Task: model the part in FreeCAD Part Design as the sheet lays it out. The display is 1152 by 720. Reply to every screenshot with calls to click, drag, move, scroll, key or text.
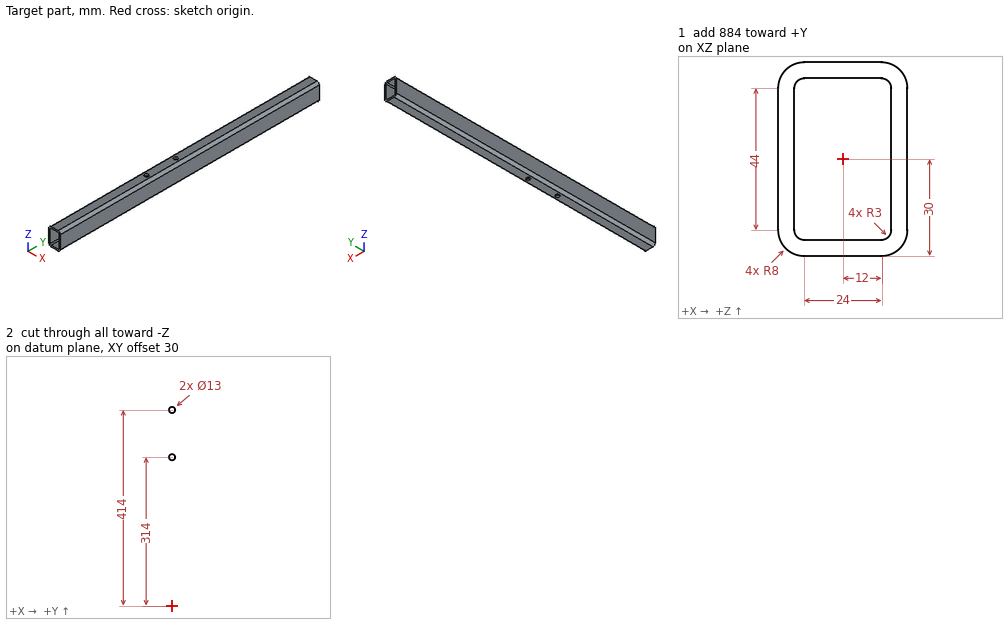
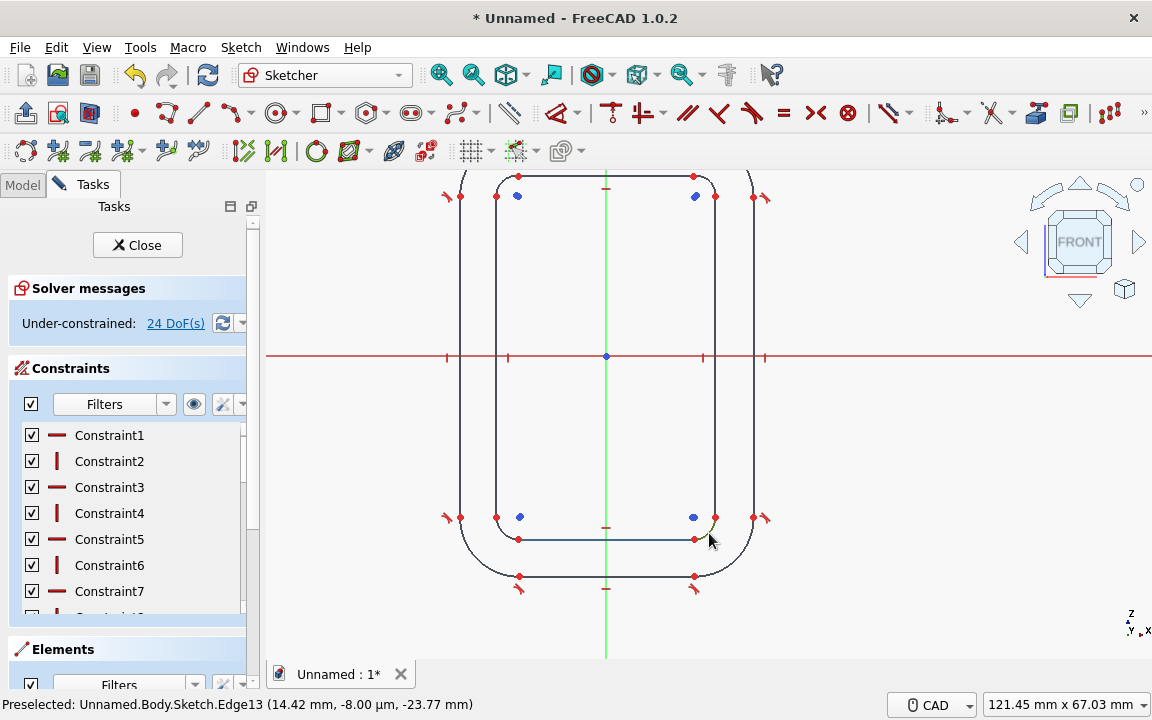
key(t)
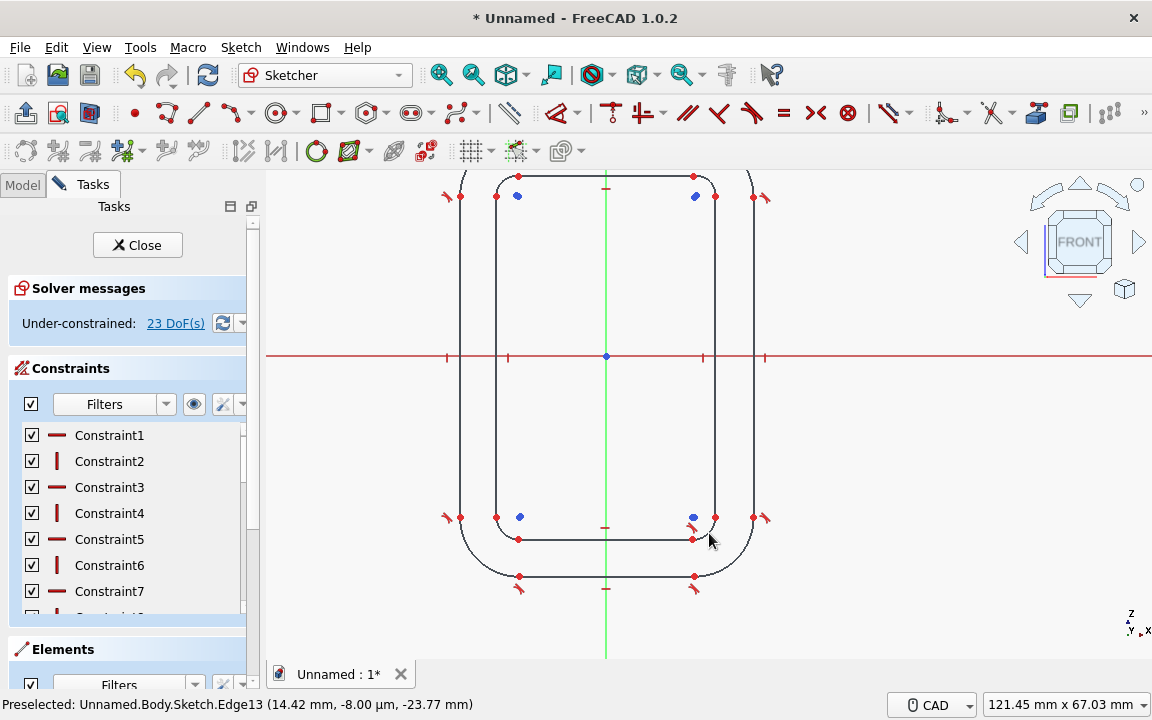
click(571, 540)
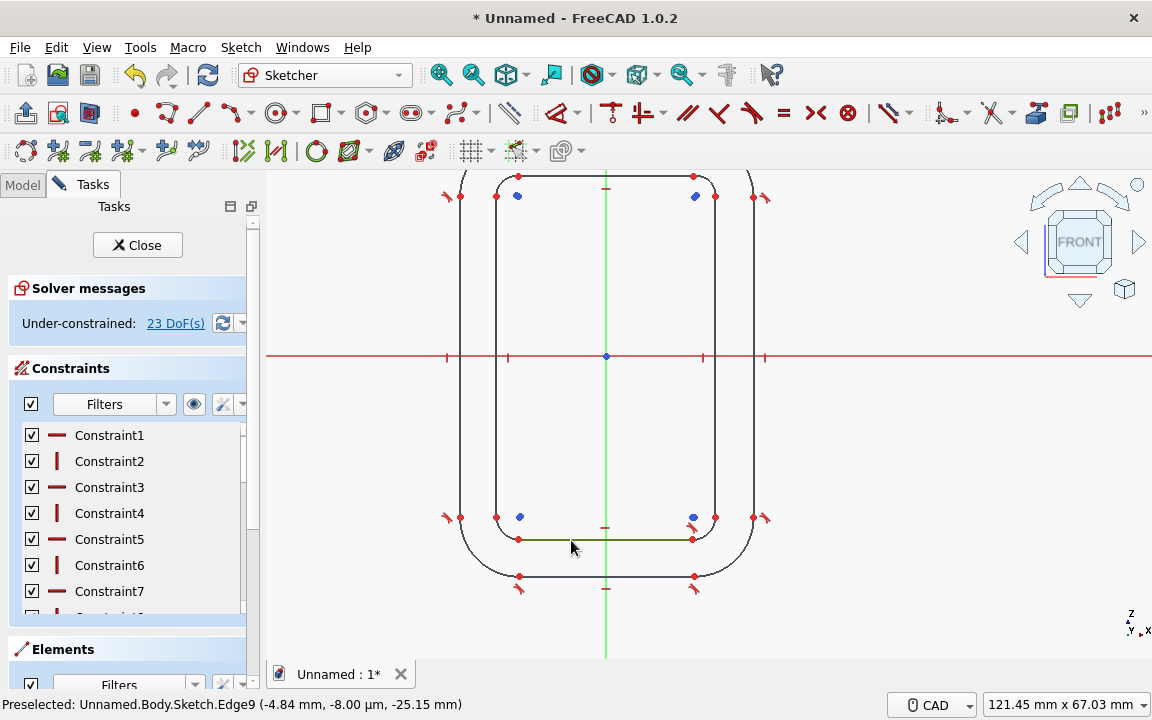
scroll(499, 527, up, 2)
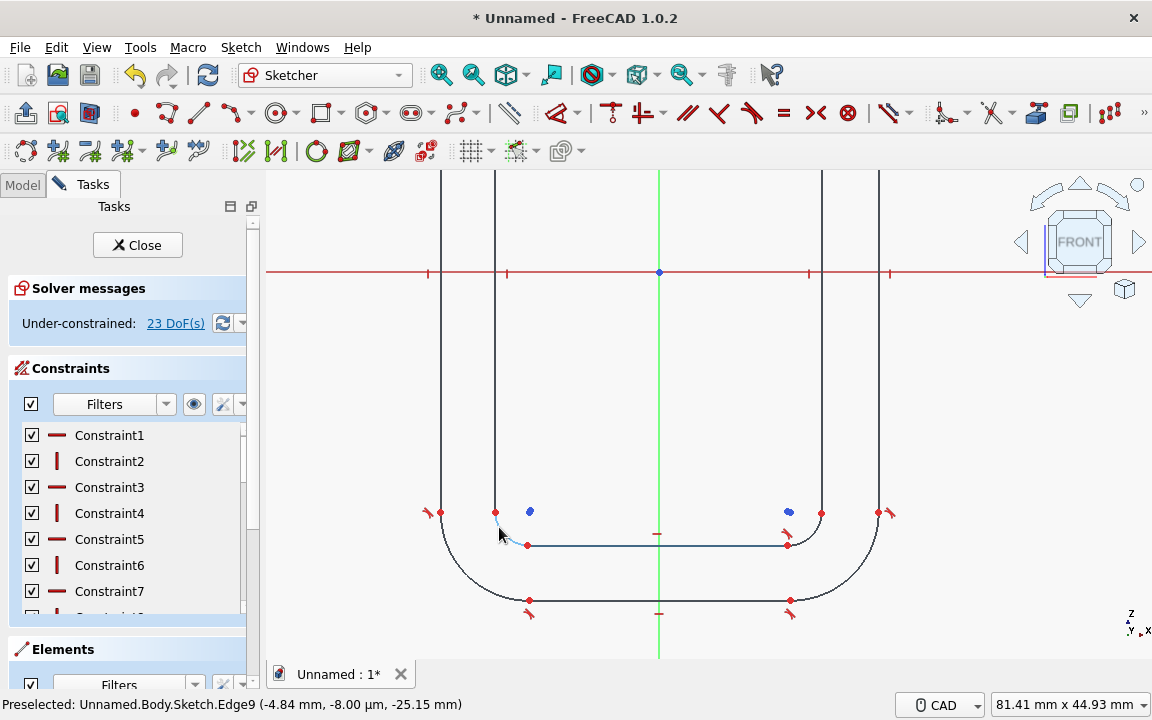
click(499, 527)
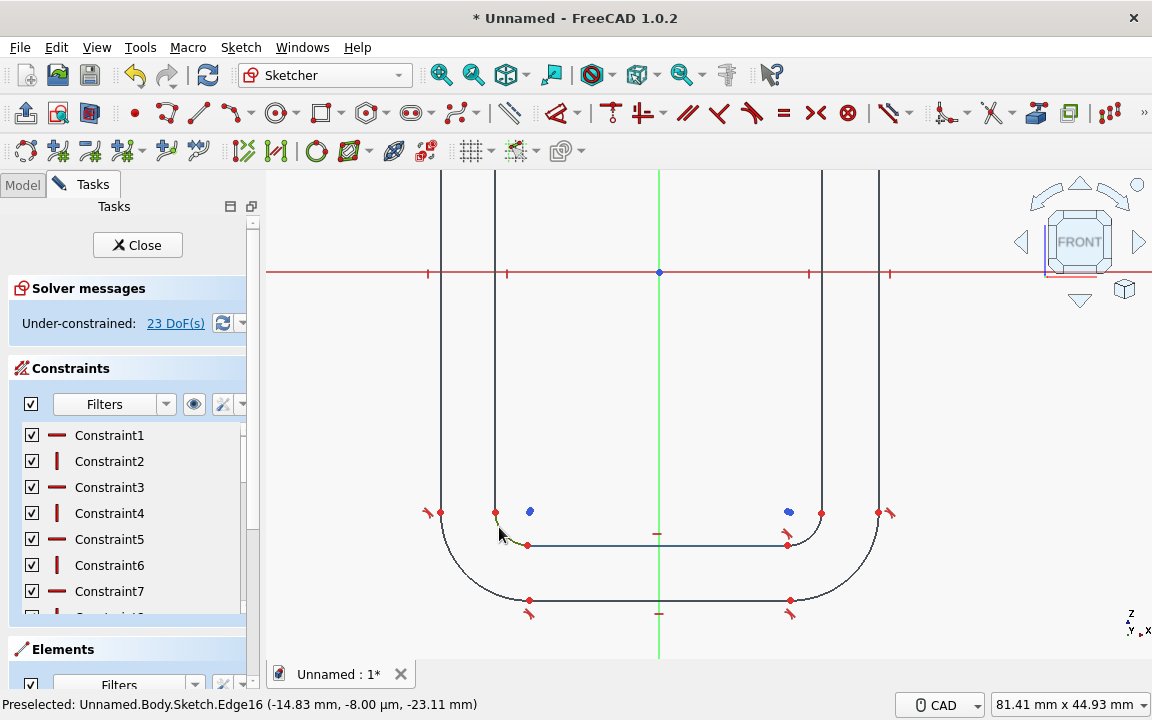
key(t)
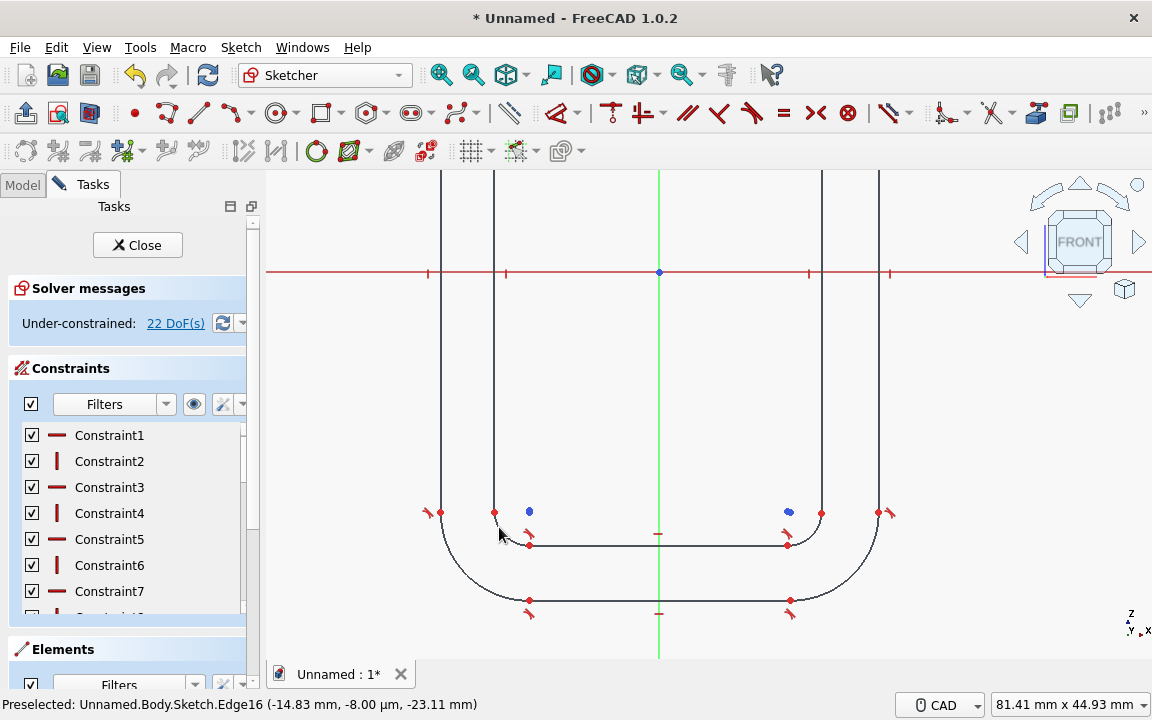
click(822, 369)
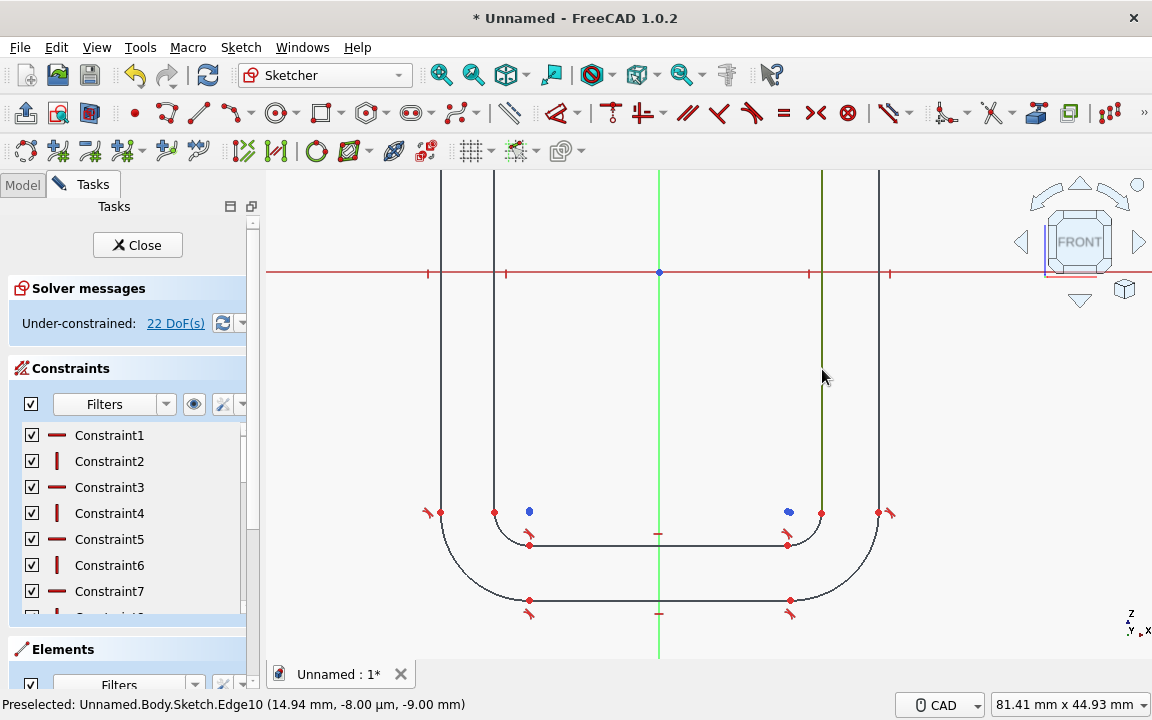
click(803, 542)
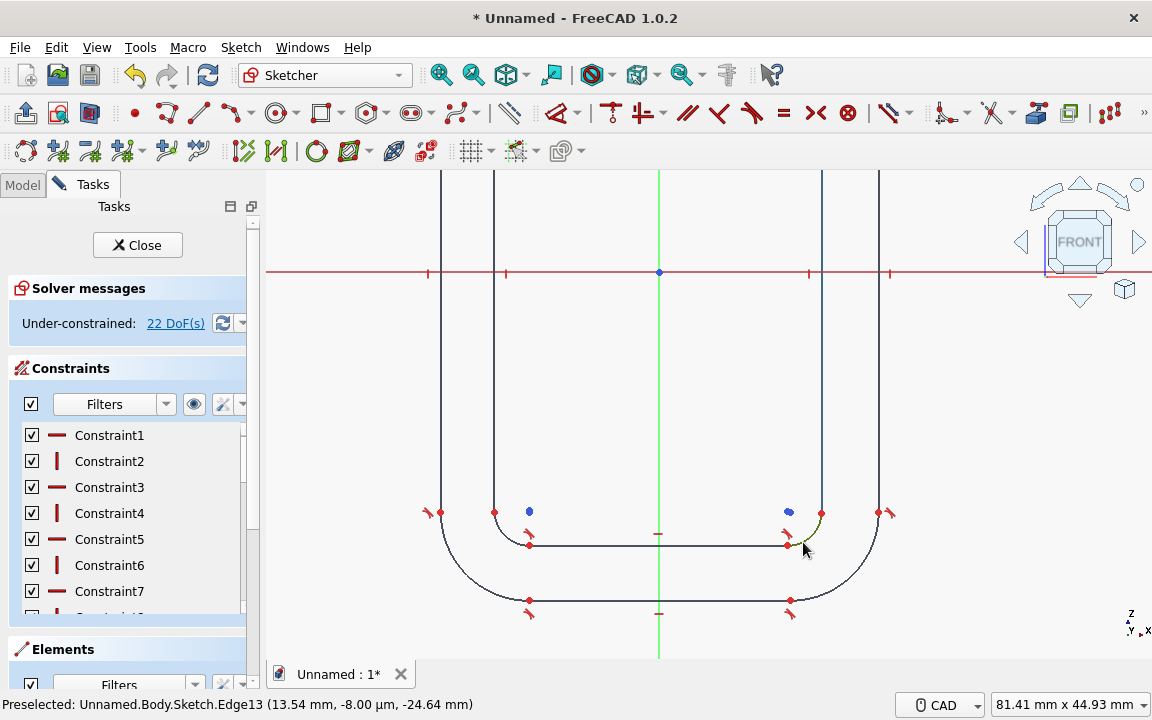
key(t)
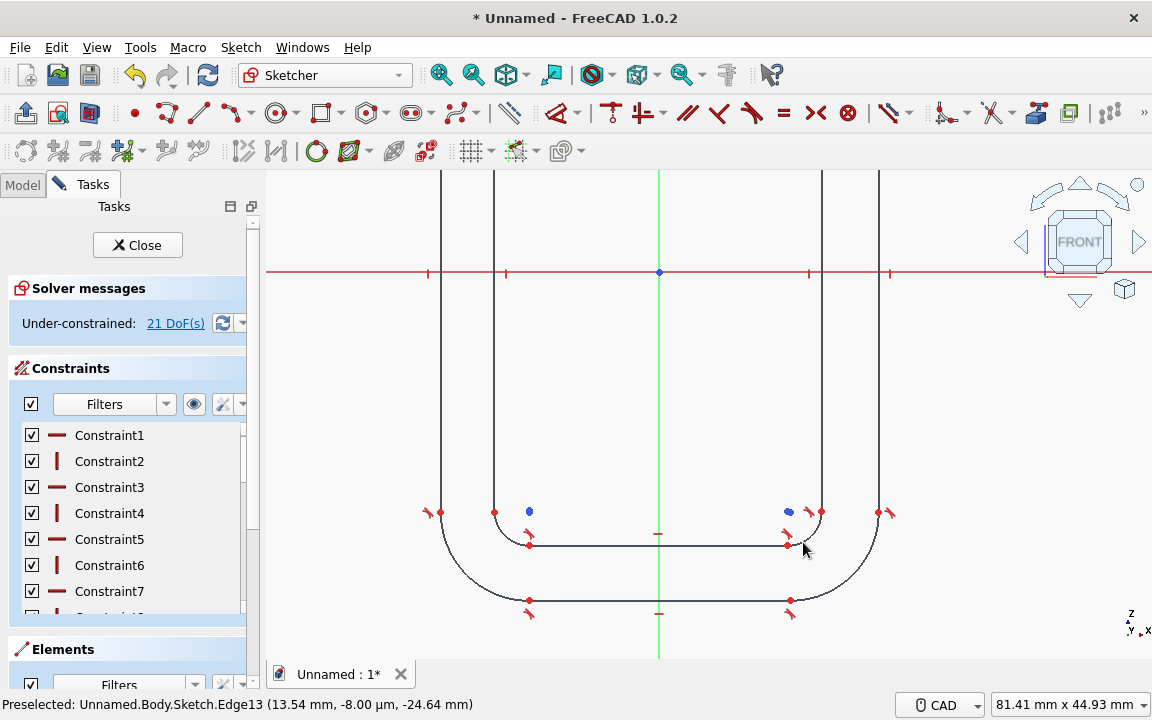
click(822, 369)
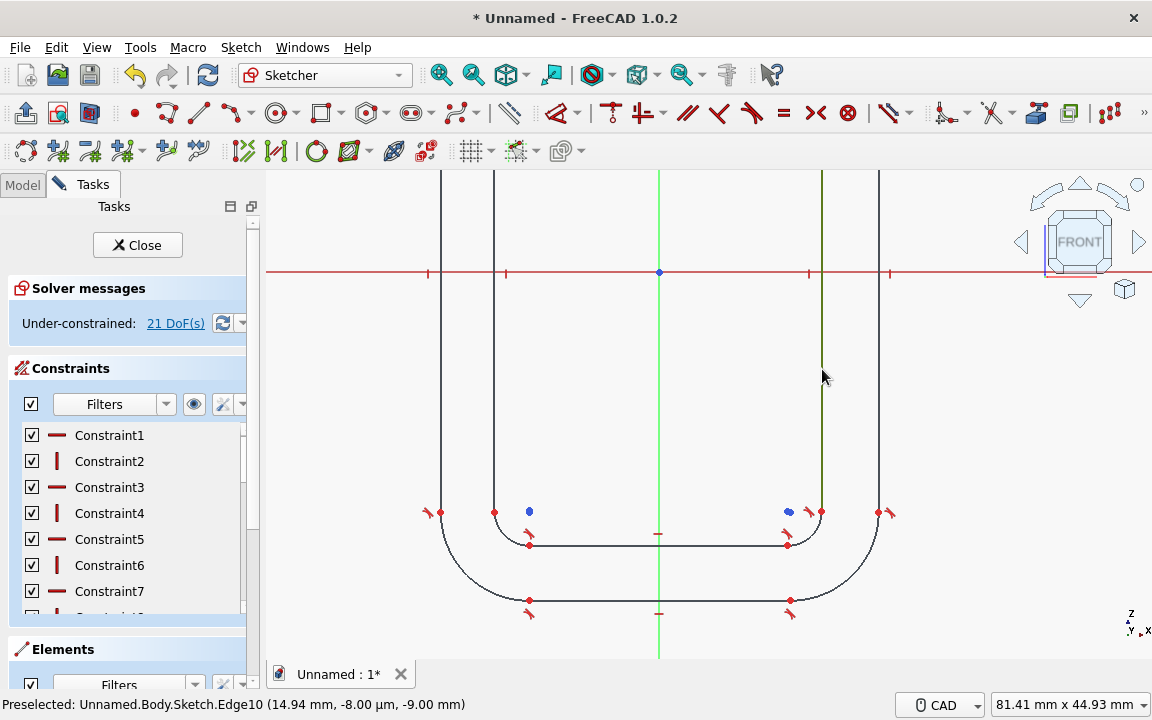
scroll(625, 531, down, 4)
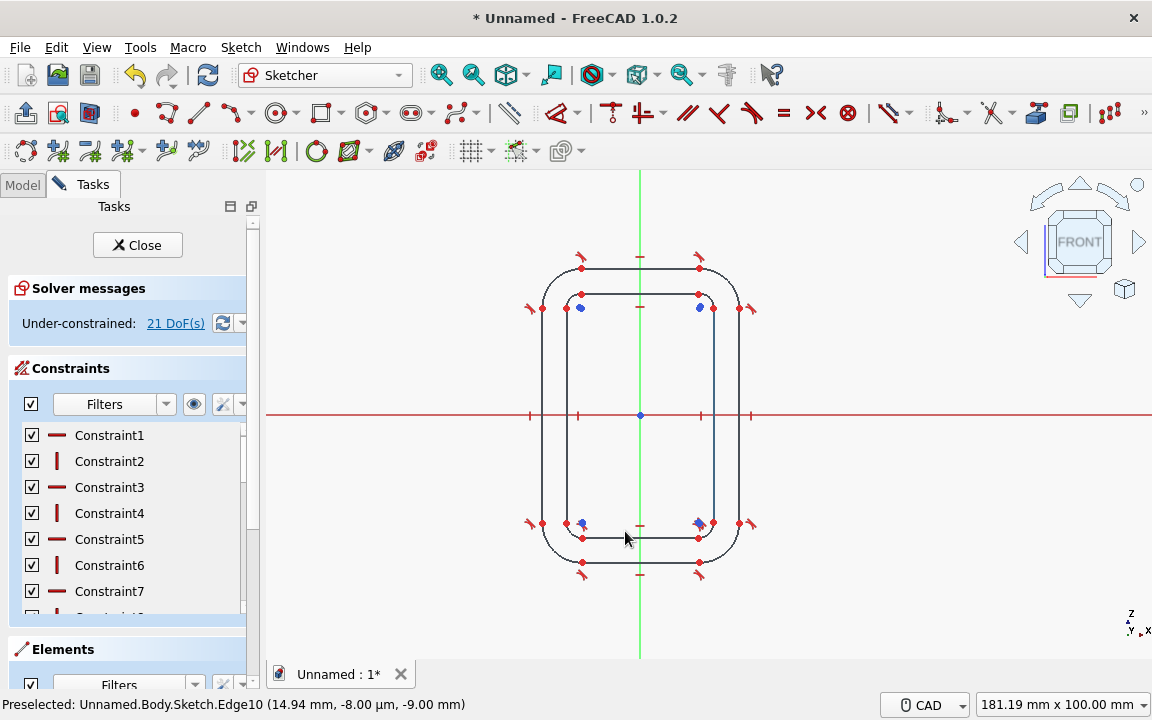
scroll(712, 301, up, 4)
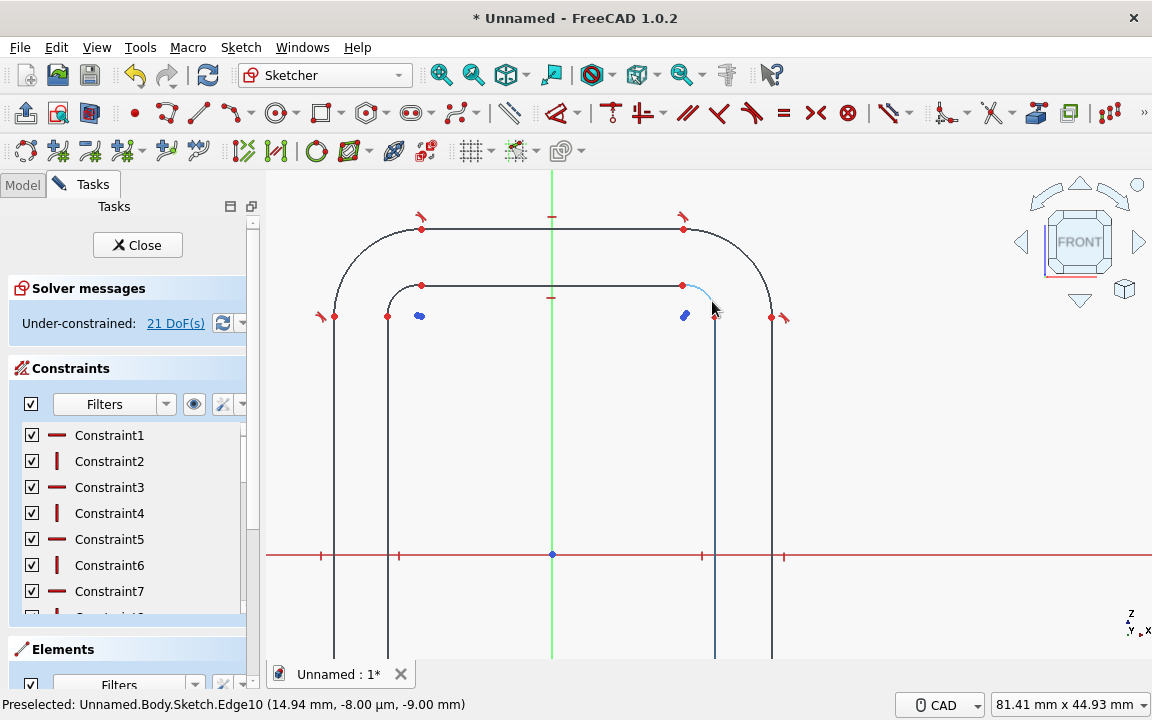
click(712, 302)